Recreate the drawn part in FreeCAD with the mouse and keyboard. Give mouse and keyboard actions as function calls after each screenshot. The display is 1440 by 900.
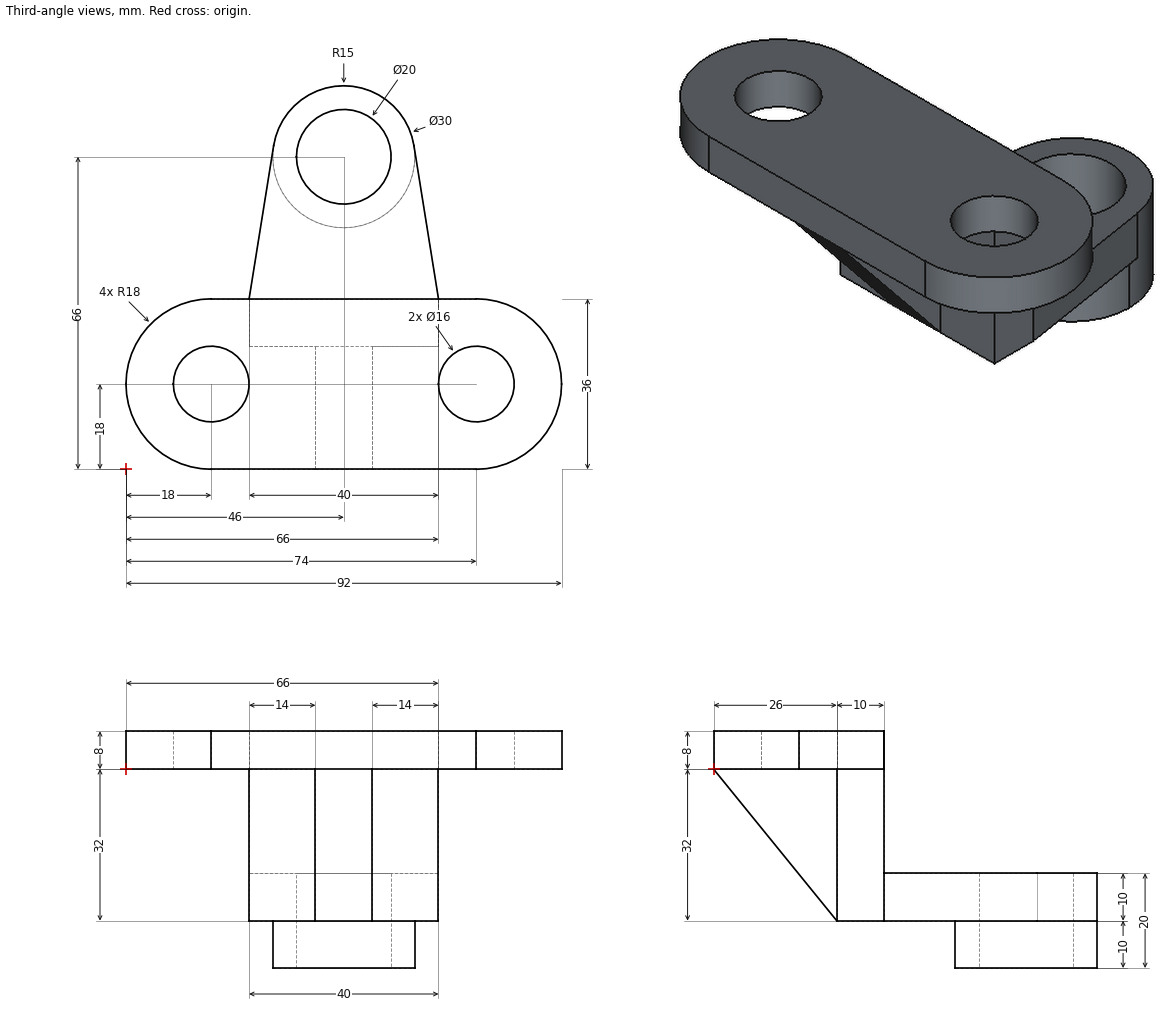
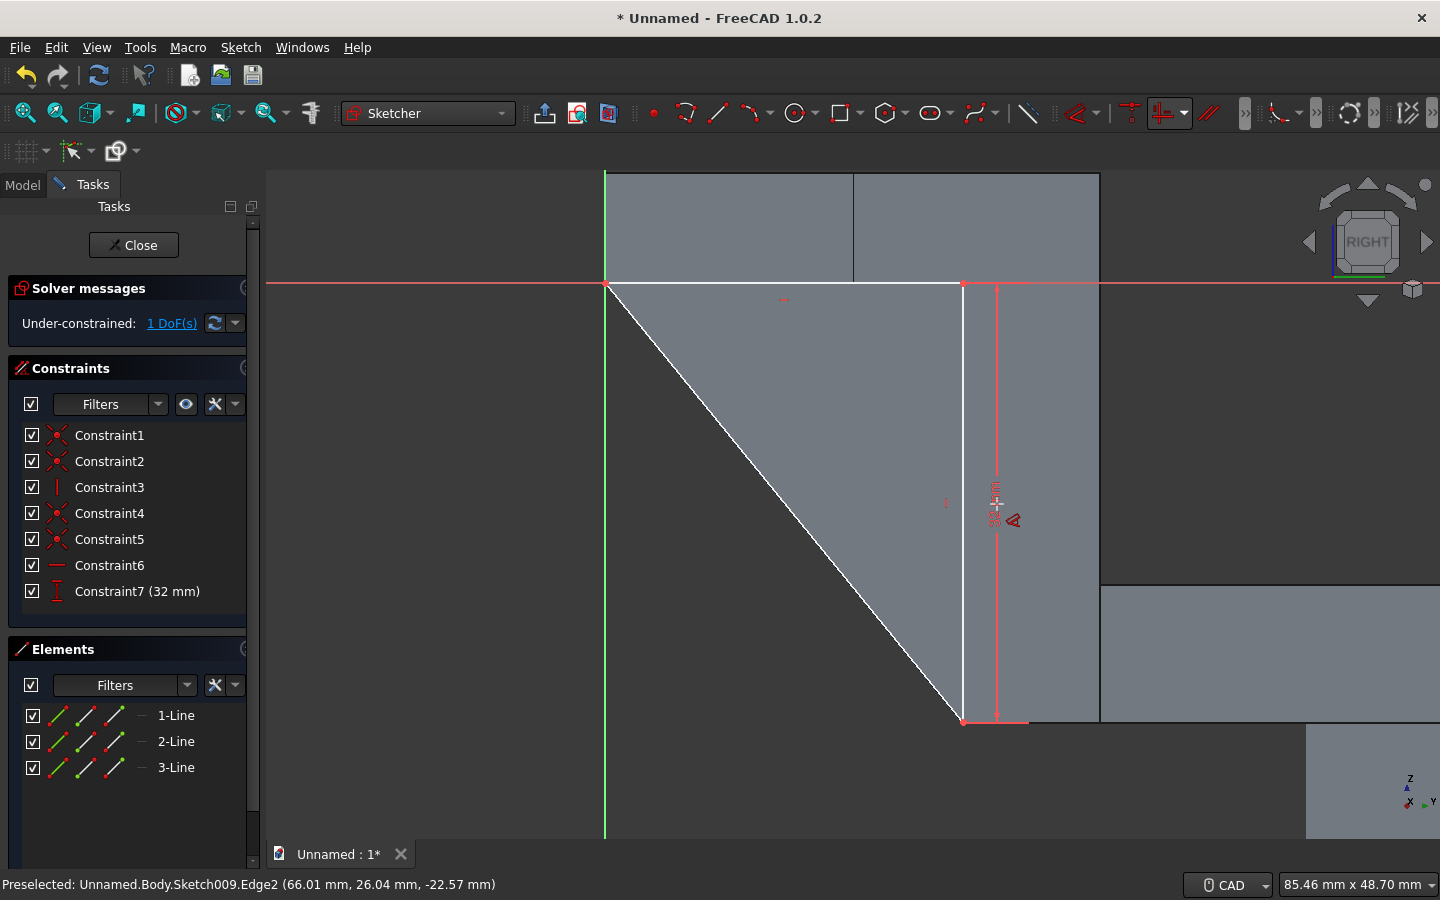
click(856, 283)
click(784, 249)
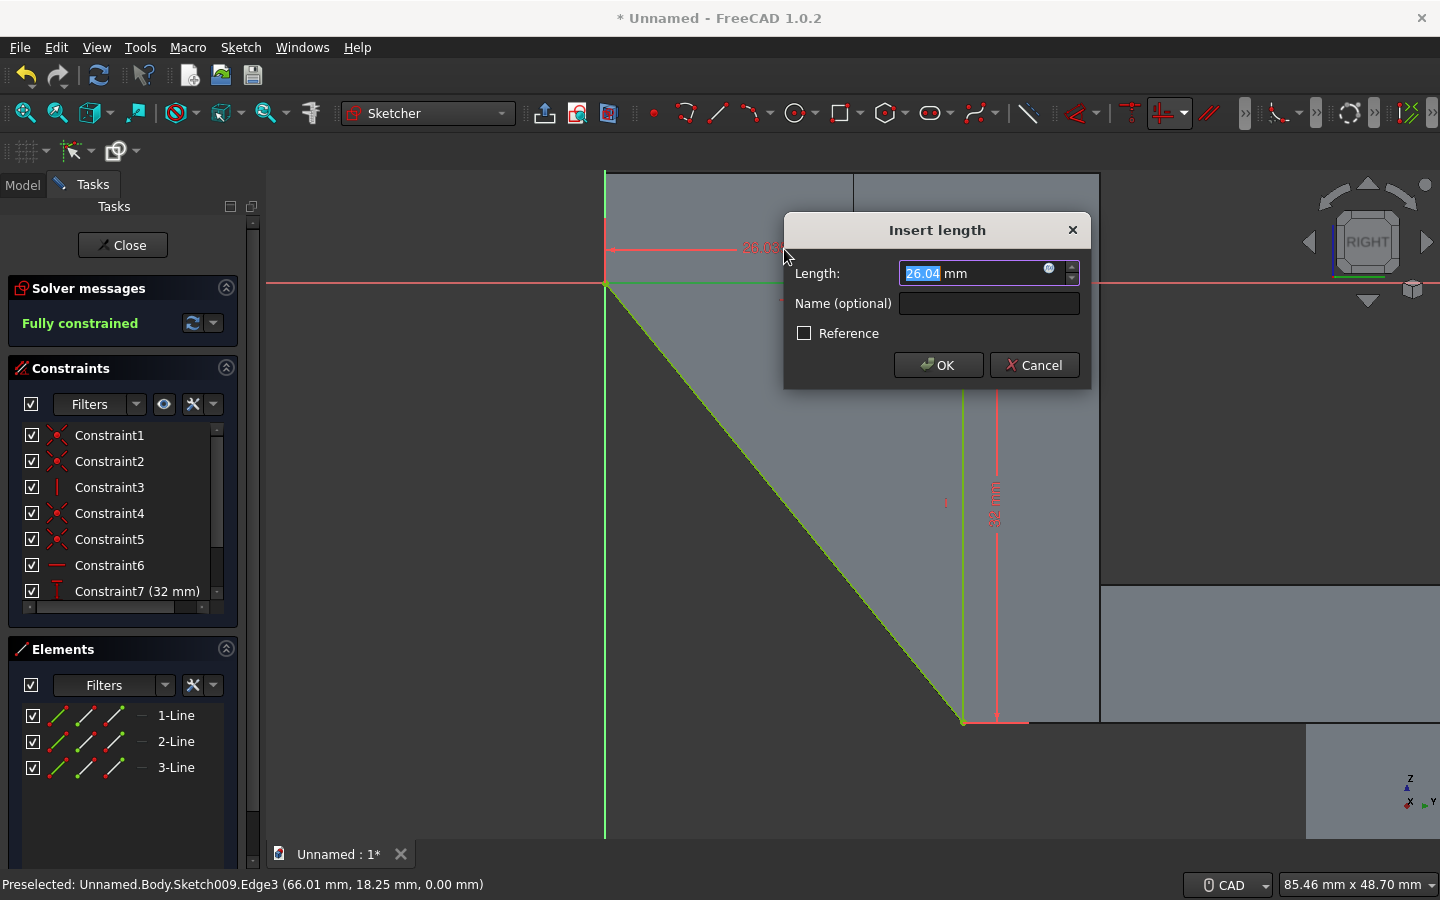
text(26)
key(Return)
key(Escape)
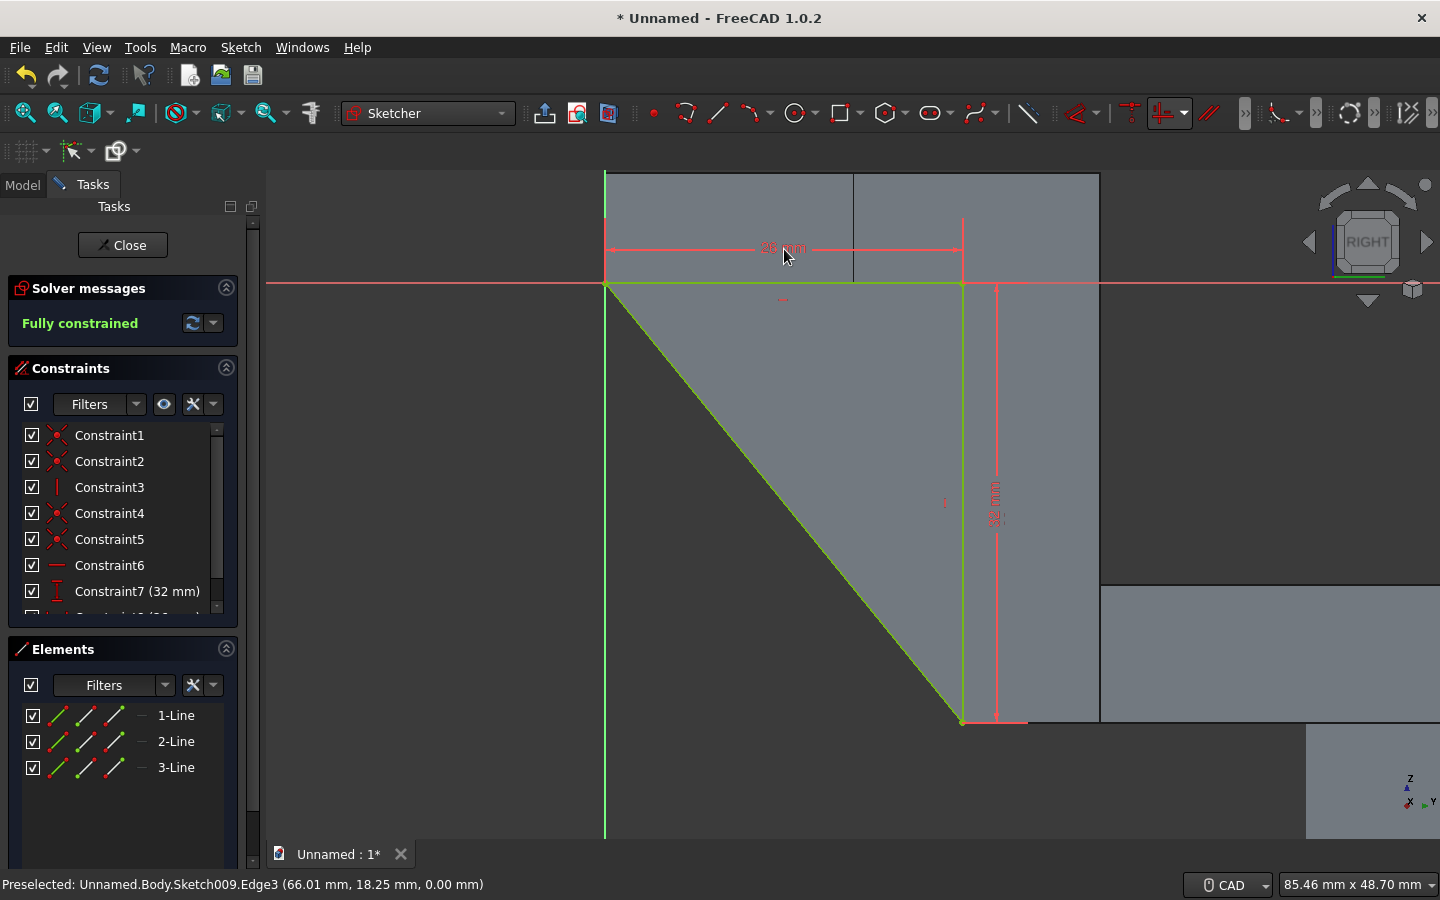
click(123, 245)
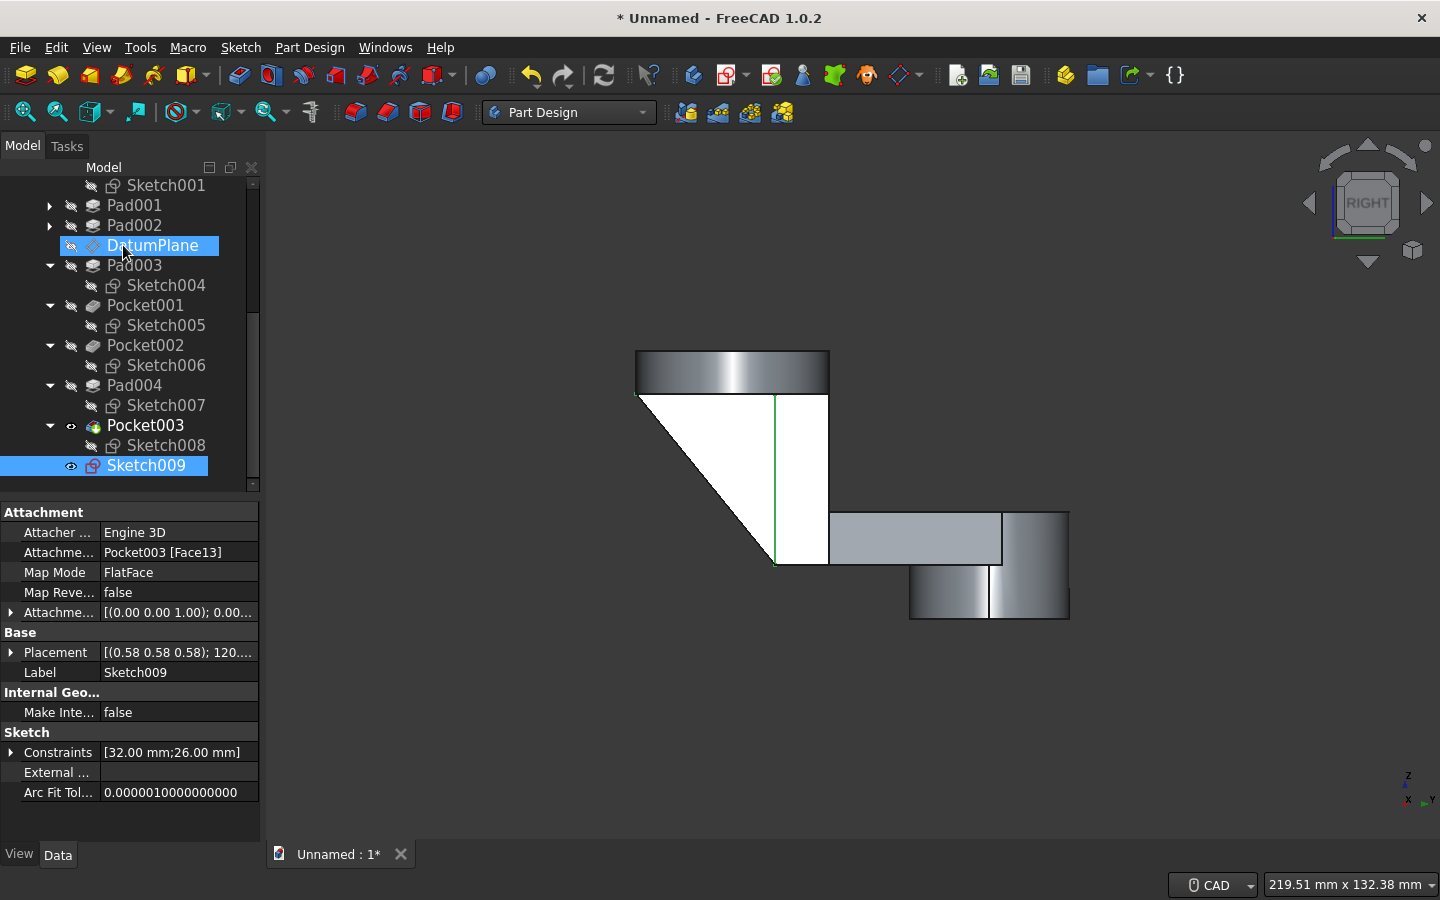
click(240, 76)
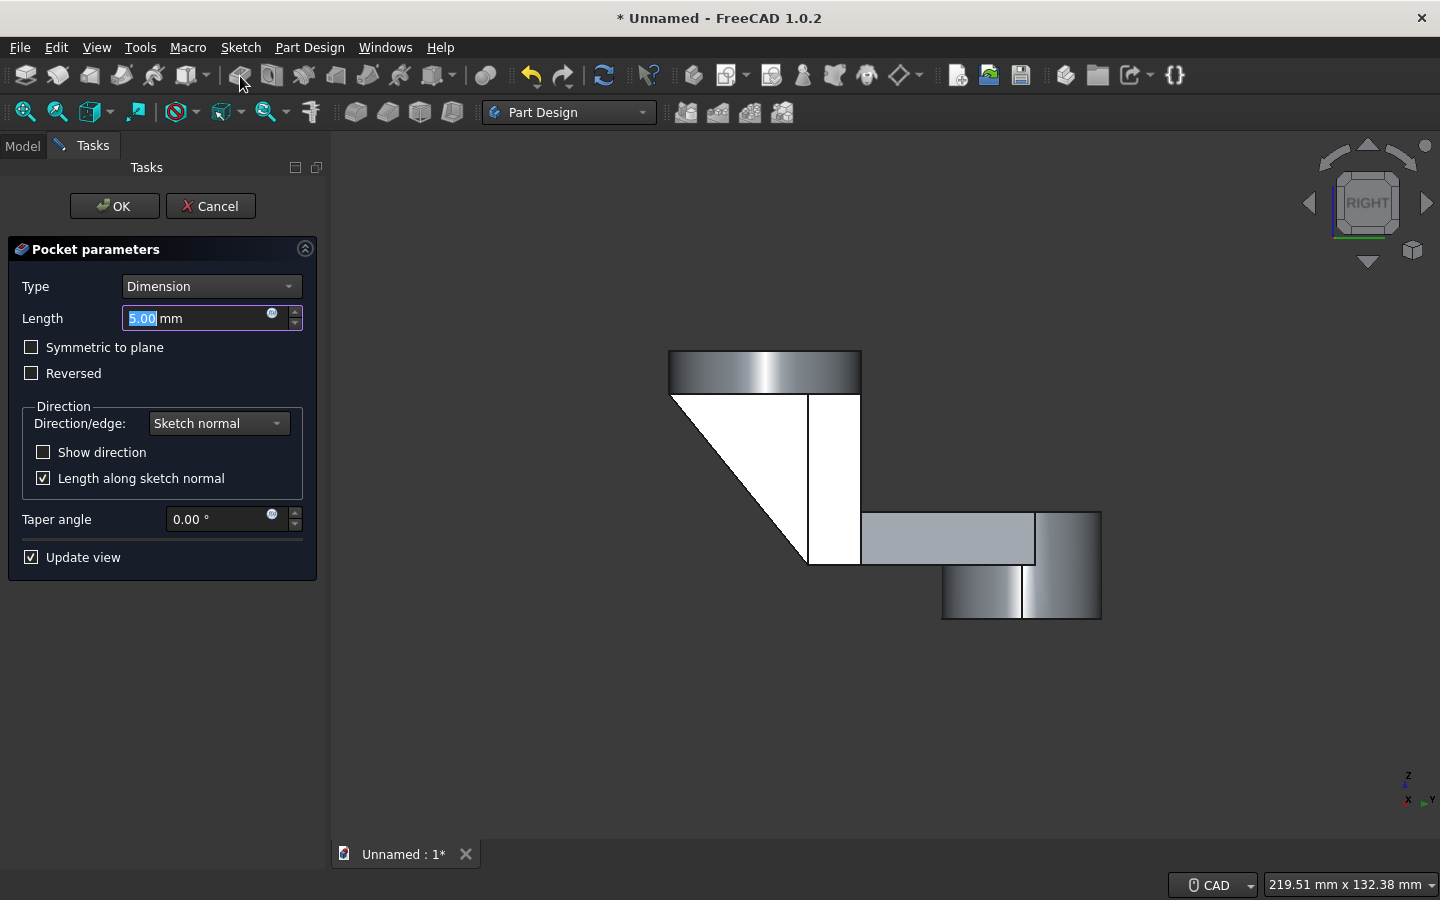
text(14)
key(Tab)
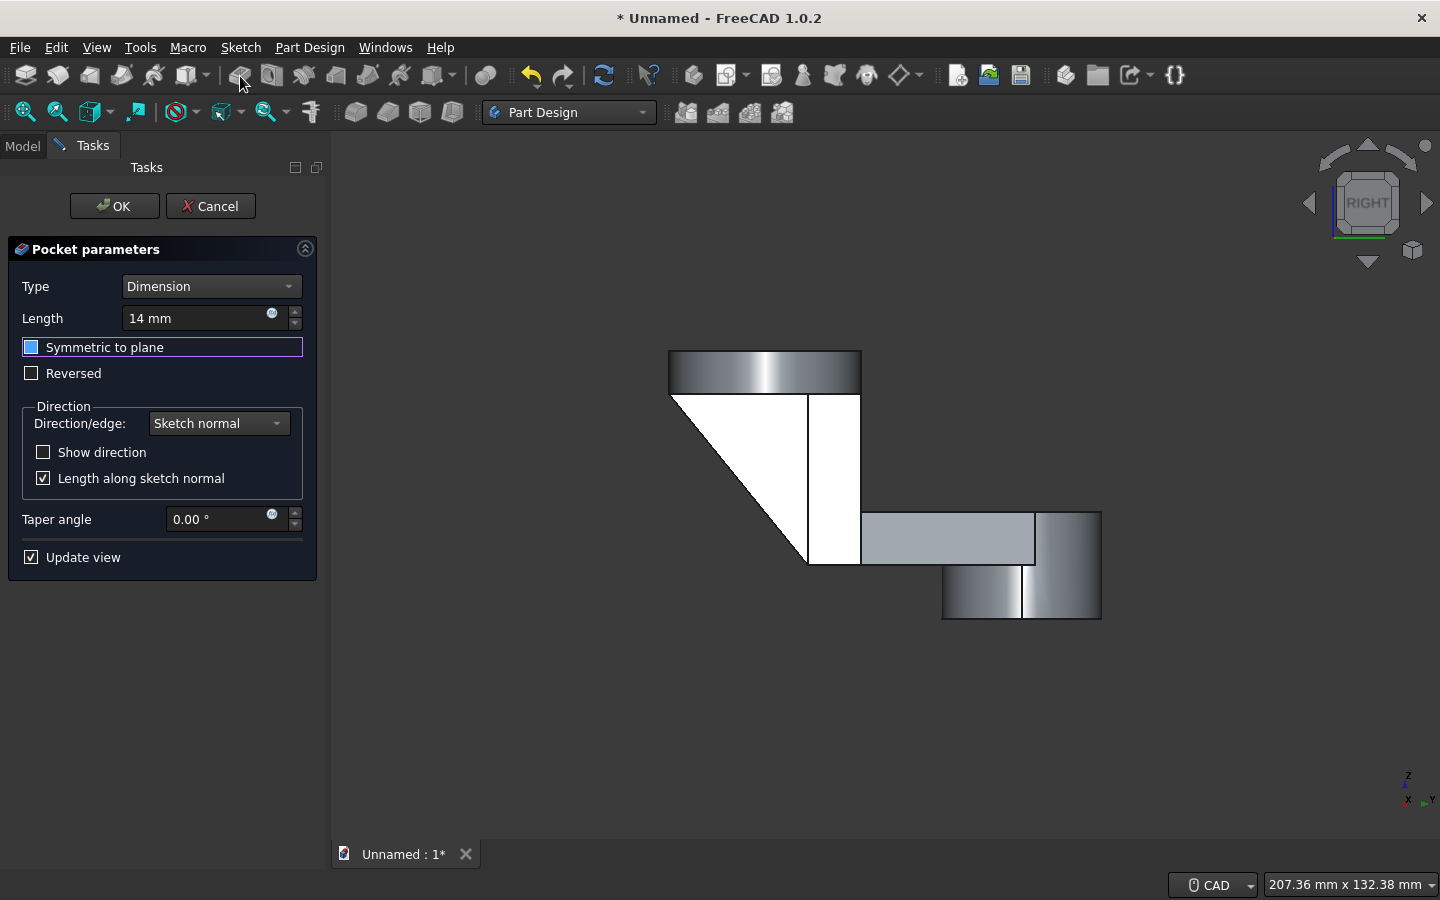
click(115, 206)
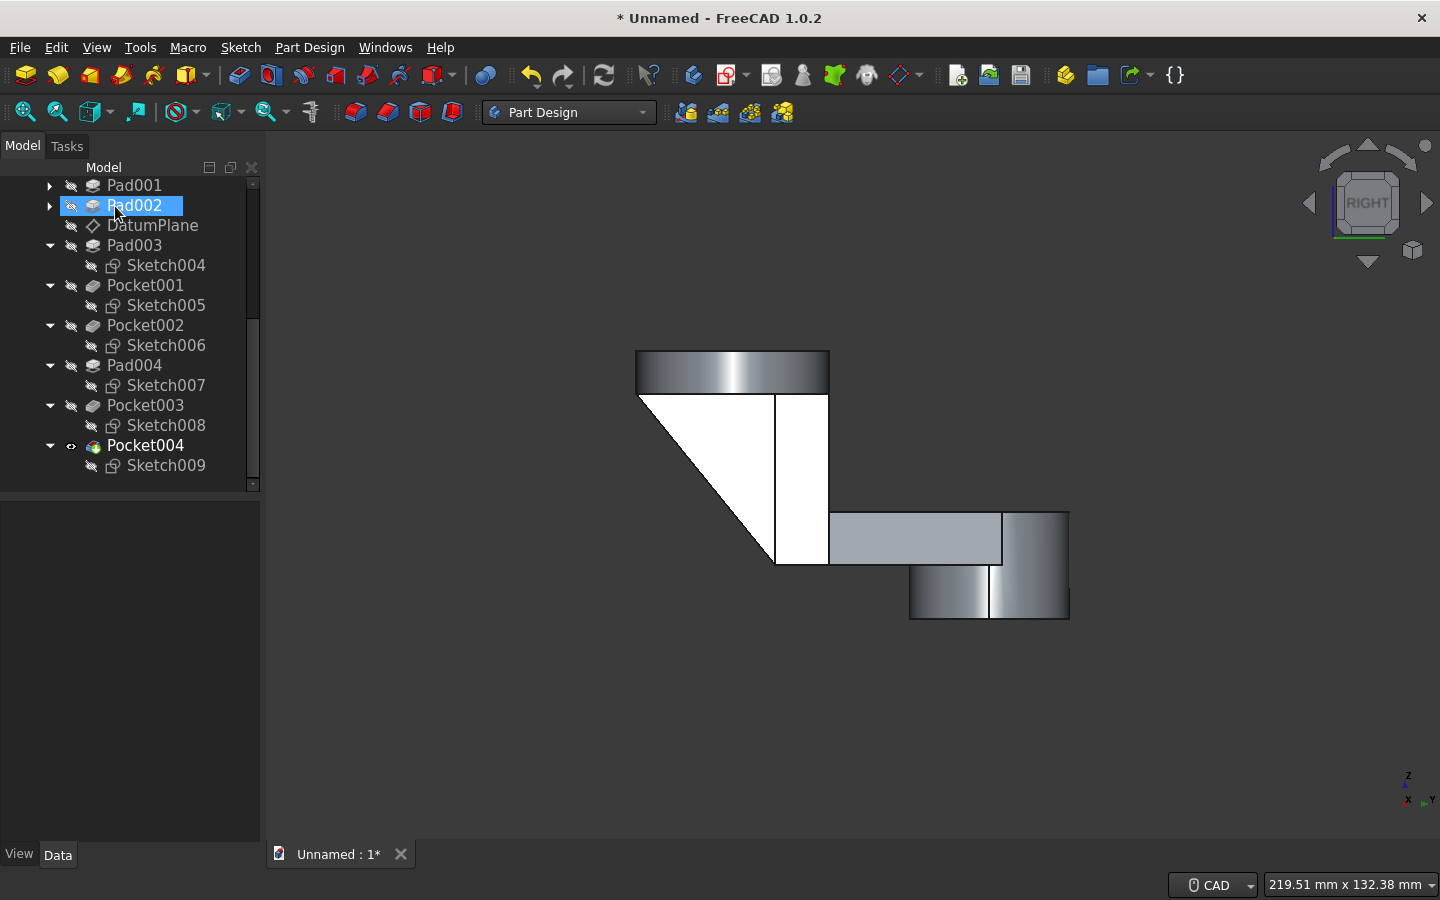
key(0)